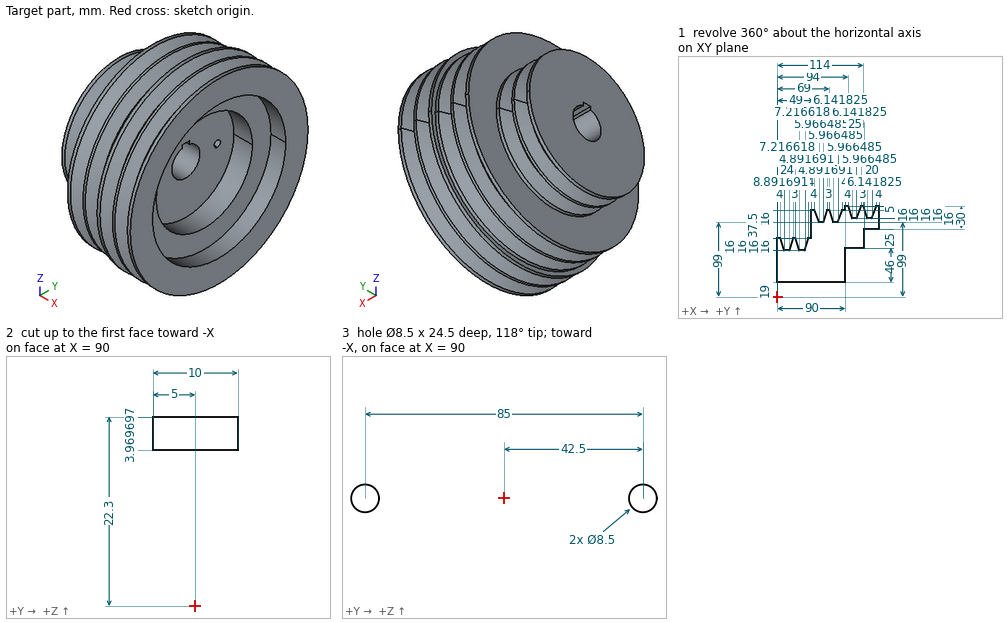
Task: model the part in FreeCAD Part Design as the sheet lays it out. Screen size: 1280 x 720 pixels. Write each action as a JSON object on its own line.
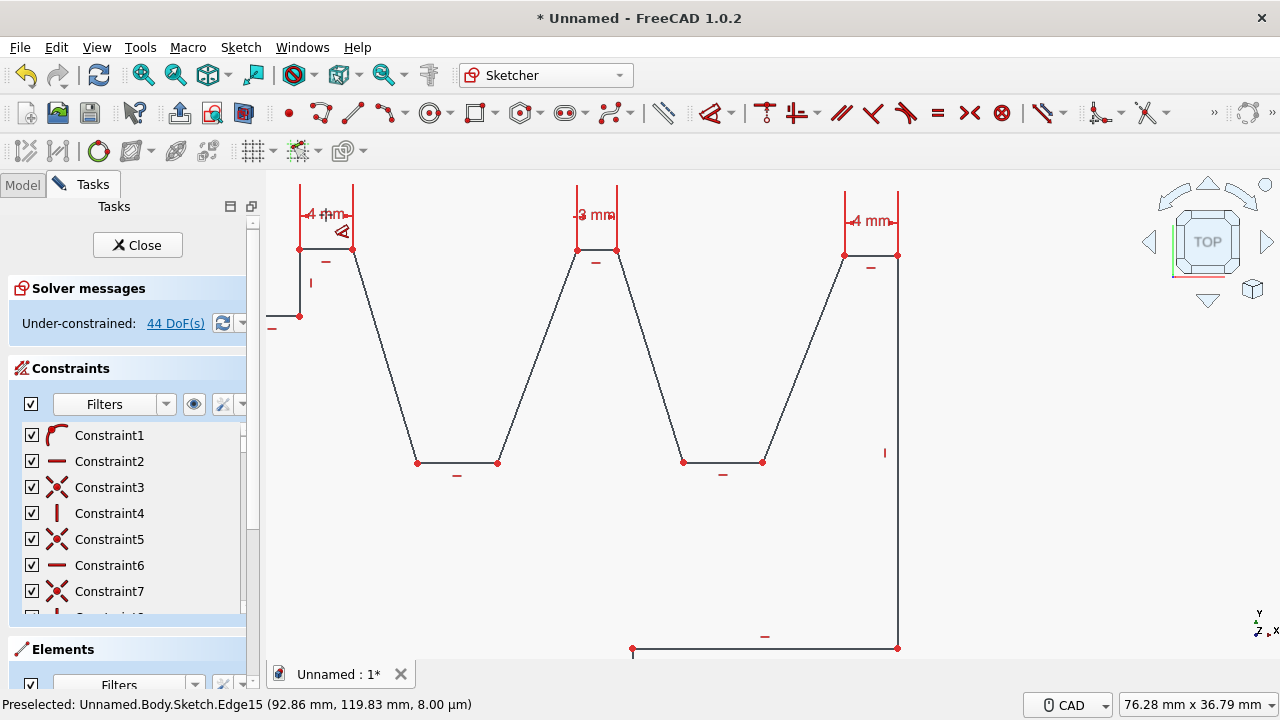
{"action": "left_click", "coordinate": [300, 269]}
{"action": "left_click", "coordinate": [334, 283]}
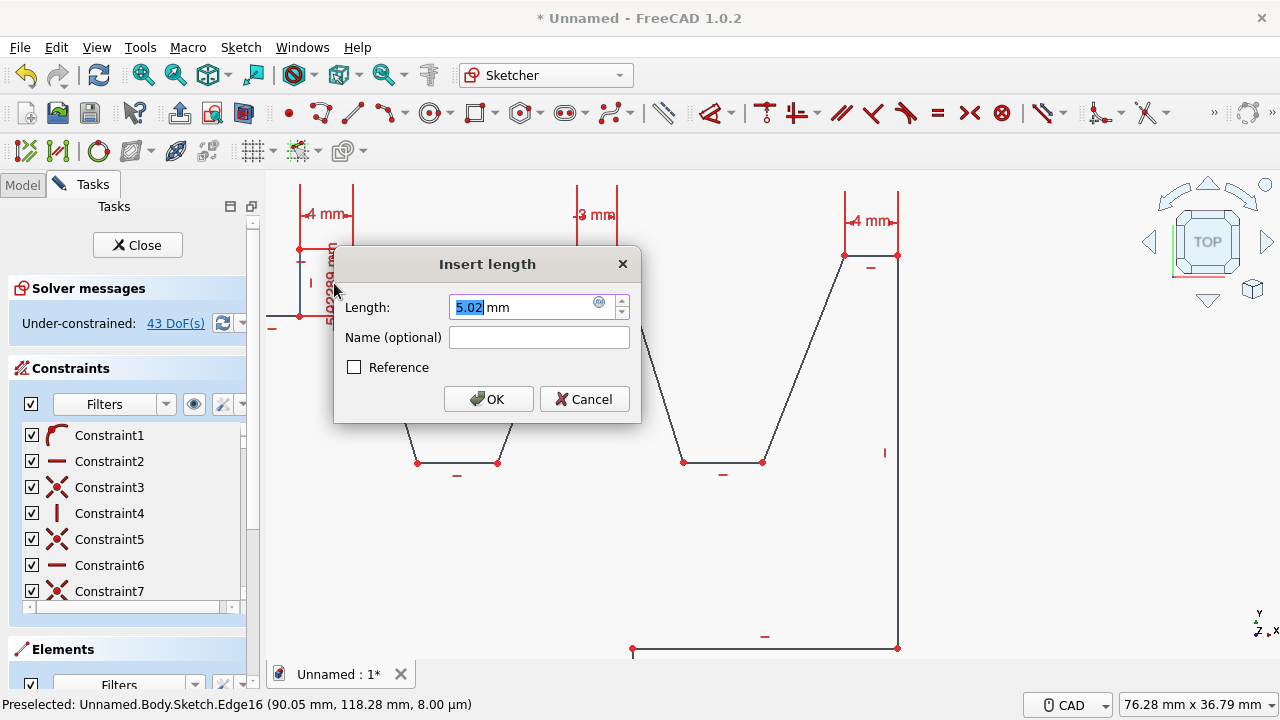
{"action": "type", "text": "5"}
{"action": "key", "text": "Return"}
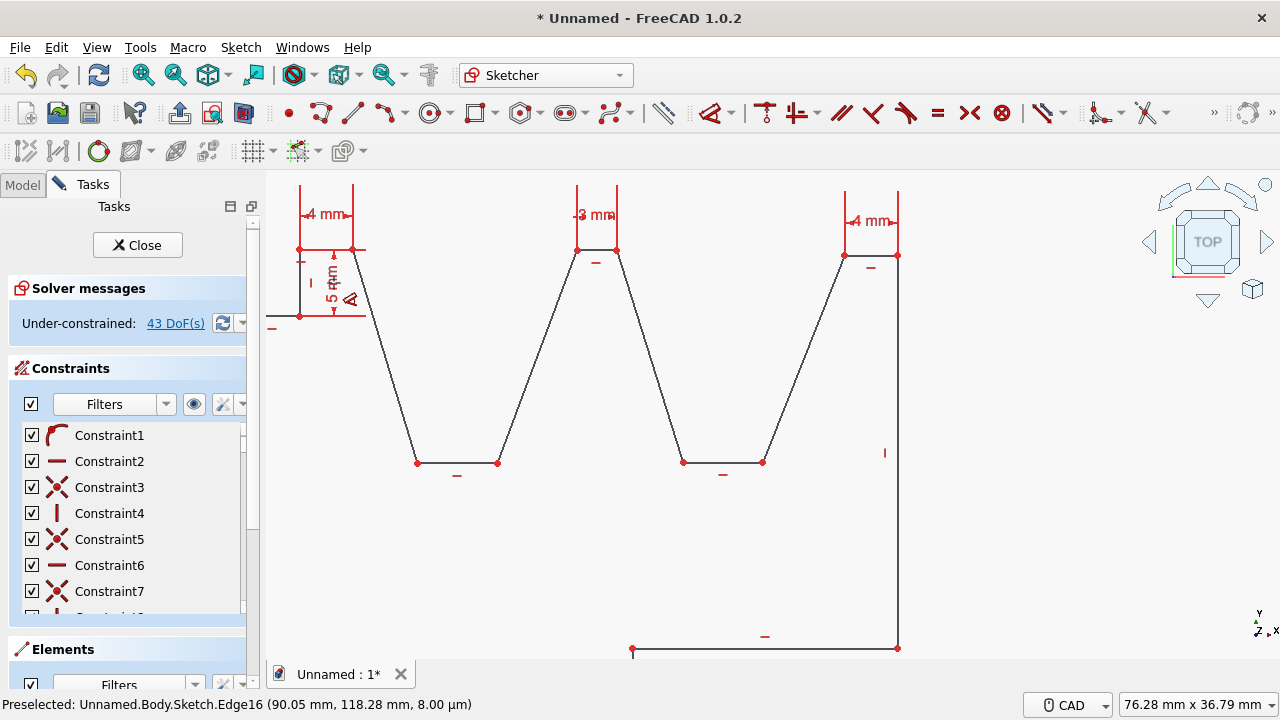
{"action": "scroll", "coordinate": [883, 255], "scroll_direction": "down", "scroll_amount": 8}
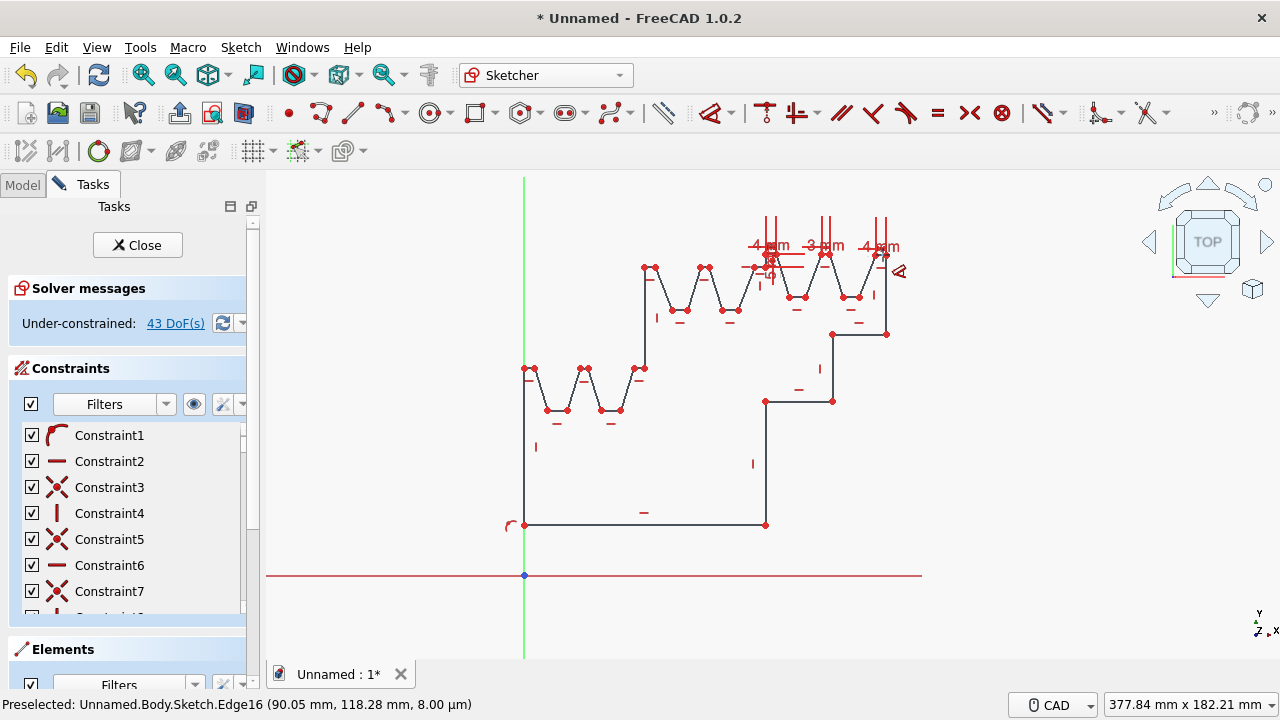
{"action": "scroll", "coordinate": [762, 267], "scroll_direction": "up", "scroll_amount": 8}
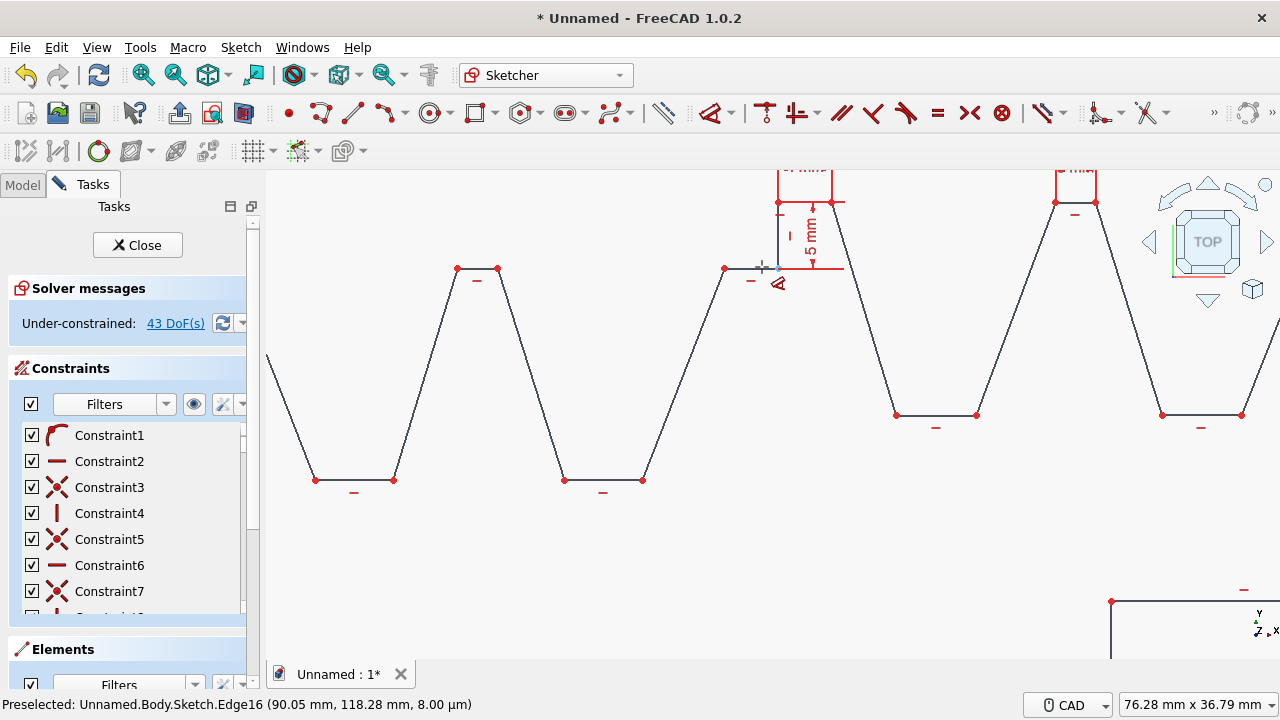
{"action": "left_click", "coordinate": [762, 269]}
{"action": "left_click", "coordinate": [739, 235]}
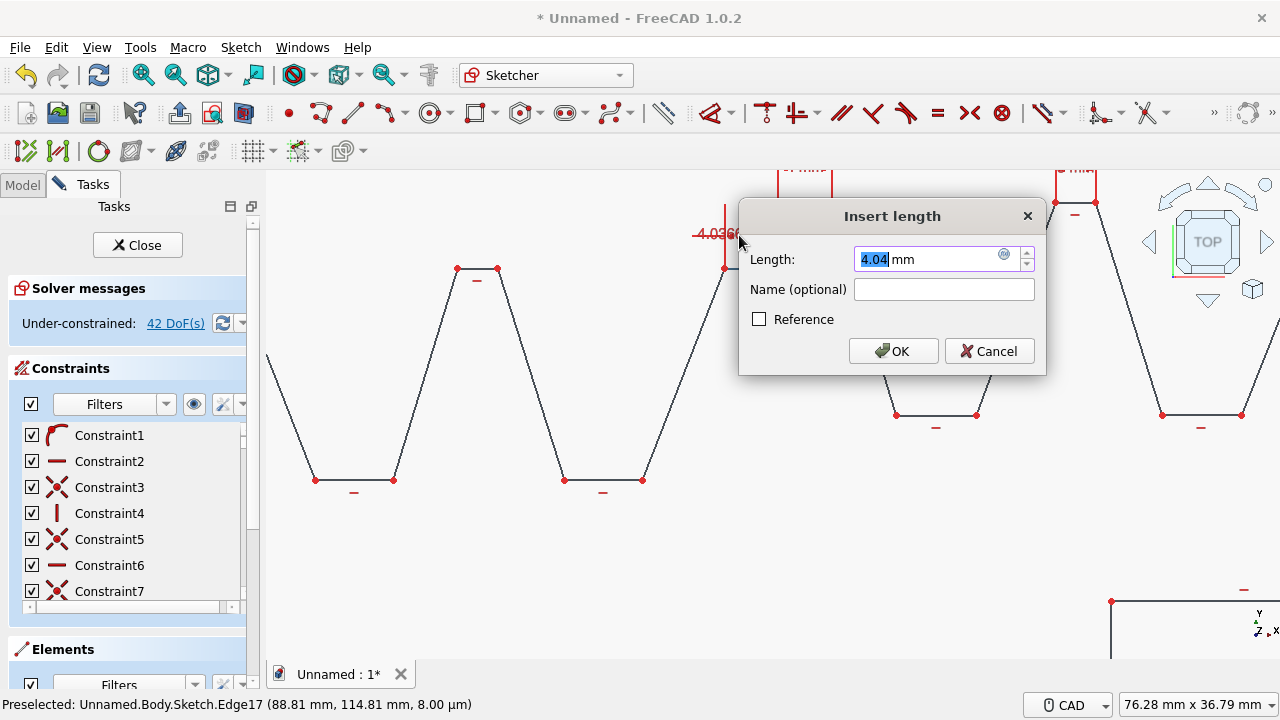
{"action": "type", "text": "4"}
{"action": "key", "text": "Return"}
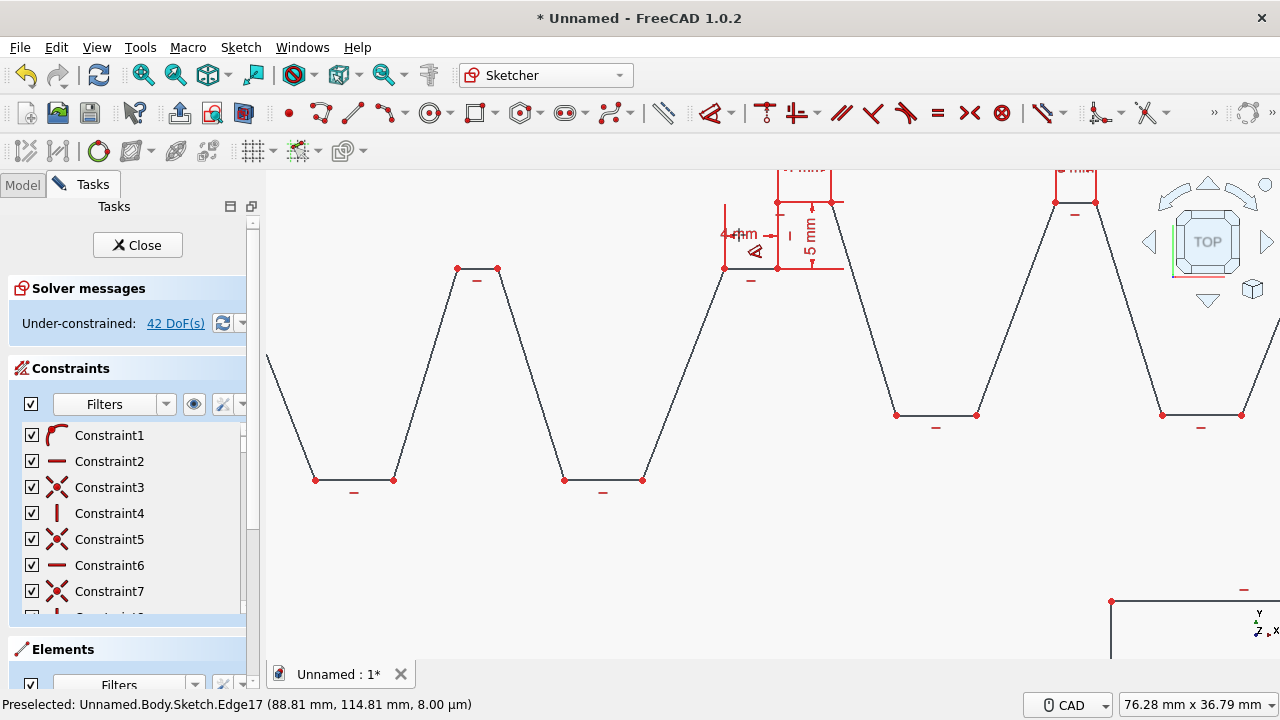
{"action": "left_click", "coordinate": [486, 269]}
{"action": "left_click", "coordinate": [478, 235]}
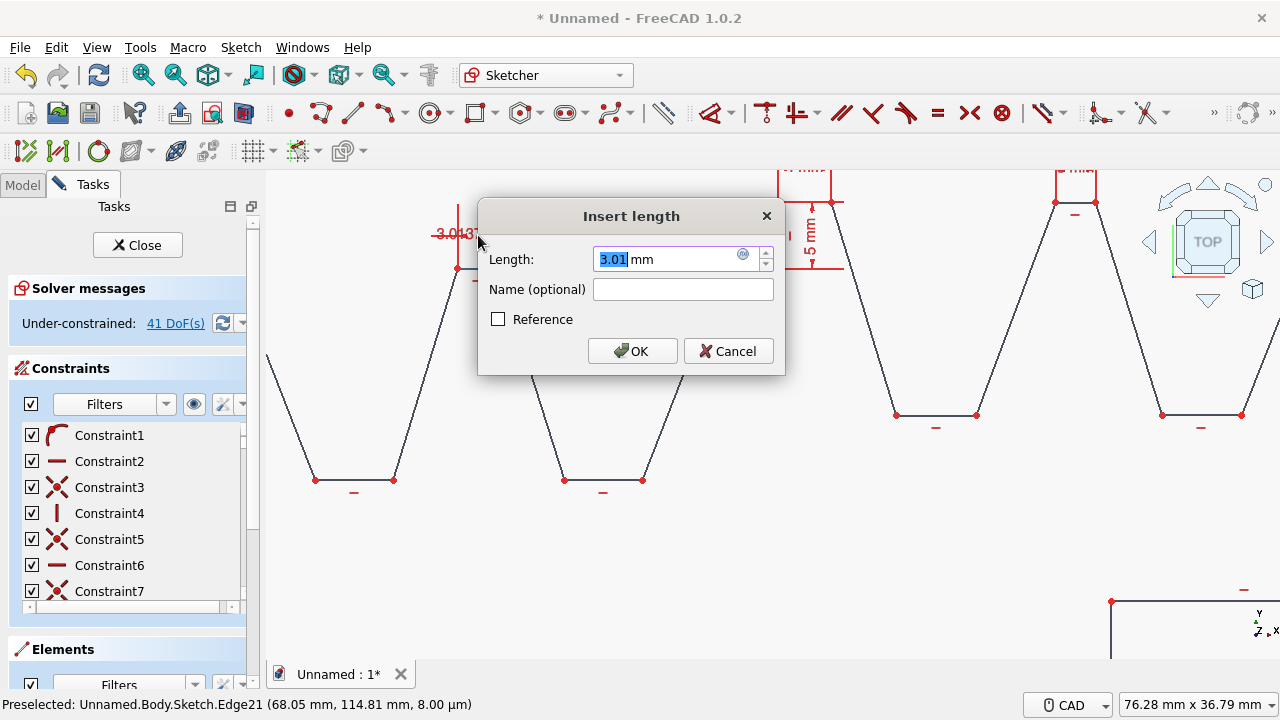
{"action": "type", "text": "3"}
{"action": "key", "text": "Return"}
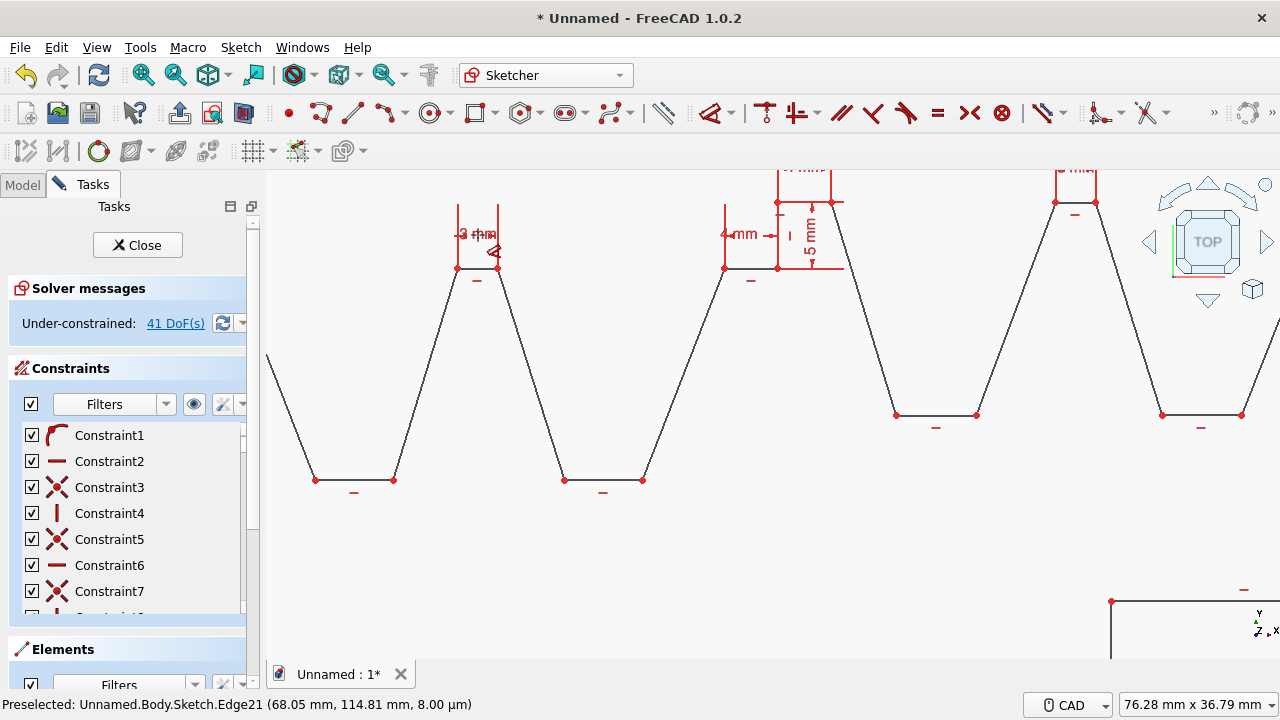
{"action": "scroll", "coordinate": [762, 267], "scroll_direction": "down", "scroll_amount": 8}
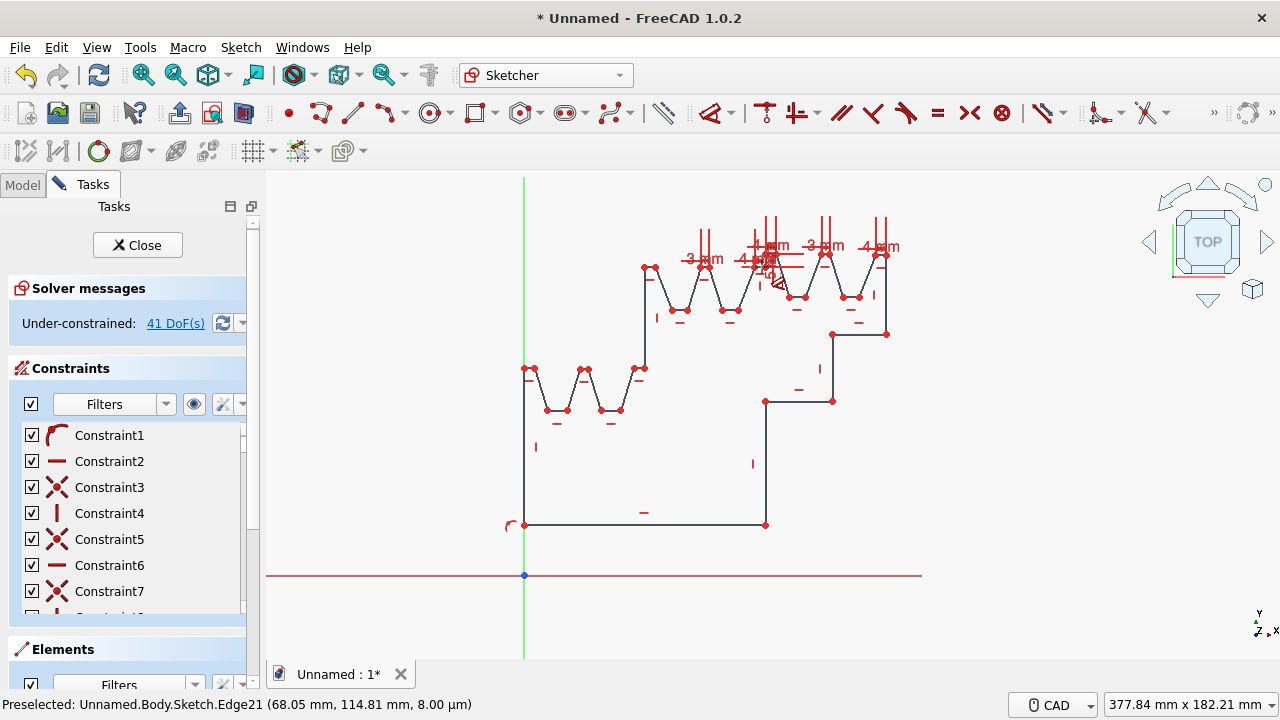
{"action": "scroll", "coordinate": [652, 267], "scroll_direction": "up", "scroll_amount": 8}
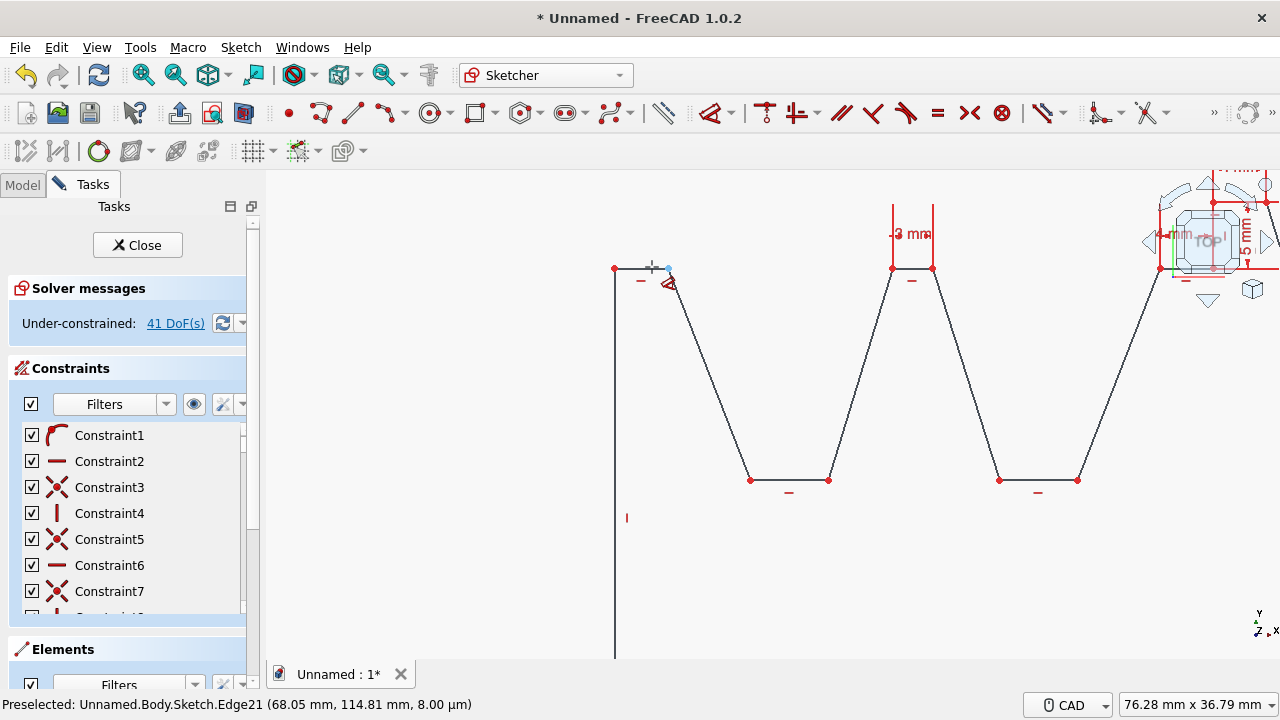
{"action": "left_click", "coordinate": [652, 269]}
{"action": "left_click", "coordinate": [641, 235]}